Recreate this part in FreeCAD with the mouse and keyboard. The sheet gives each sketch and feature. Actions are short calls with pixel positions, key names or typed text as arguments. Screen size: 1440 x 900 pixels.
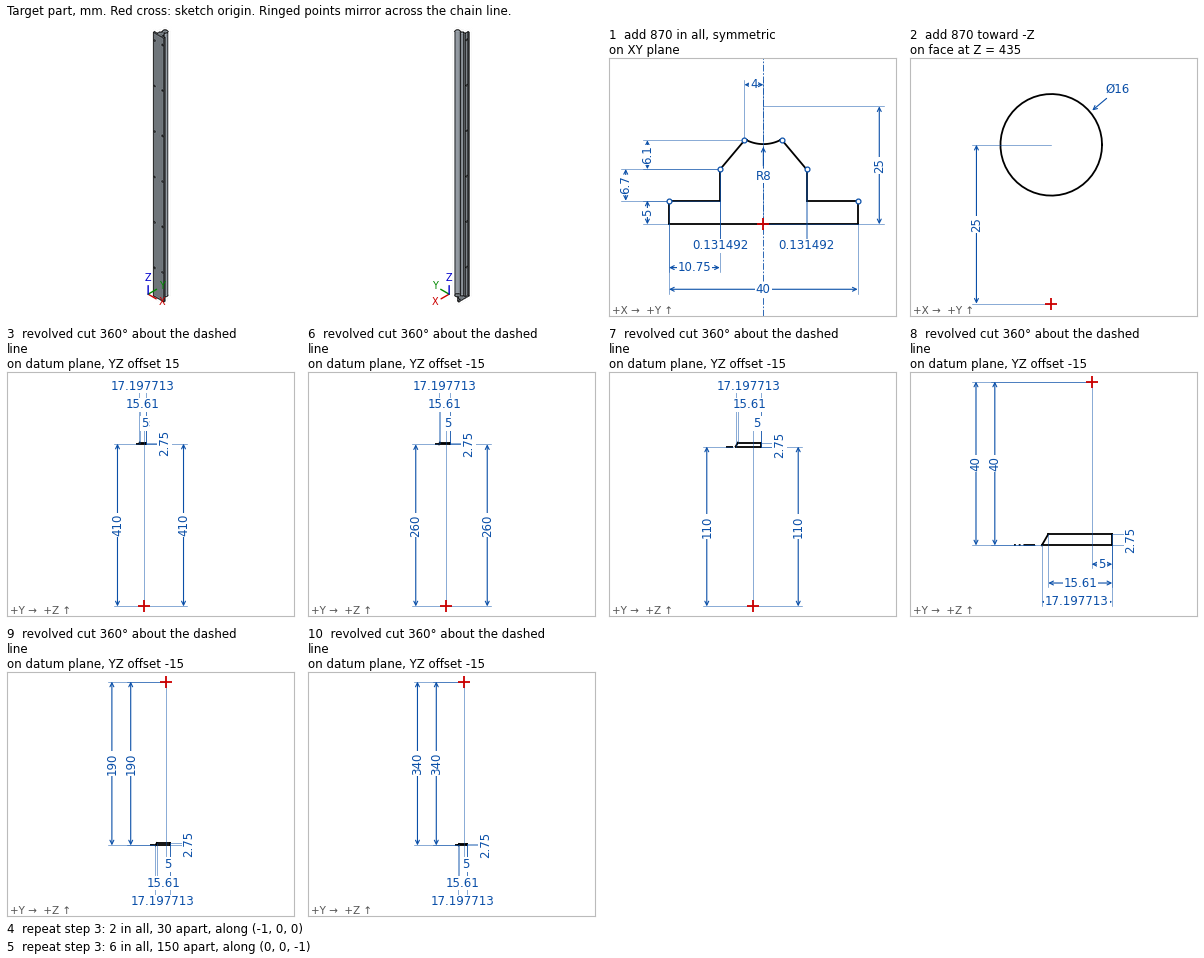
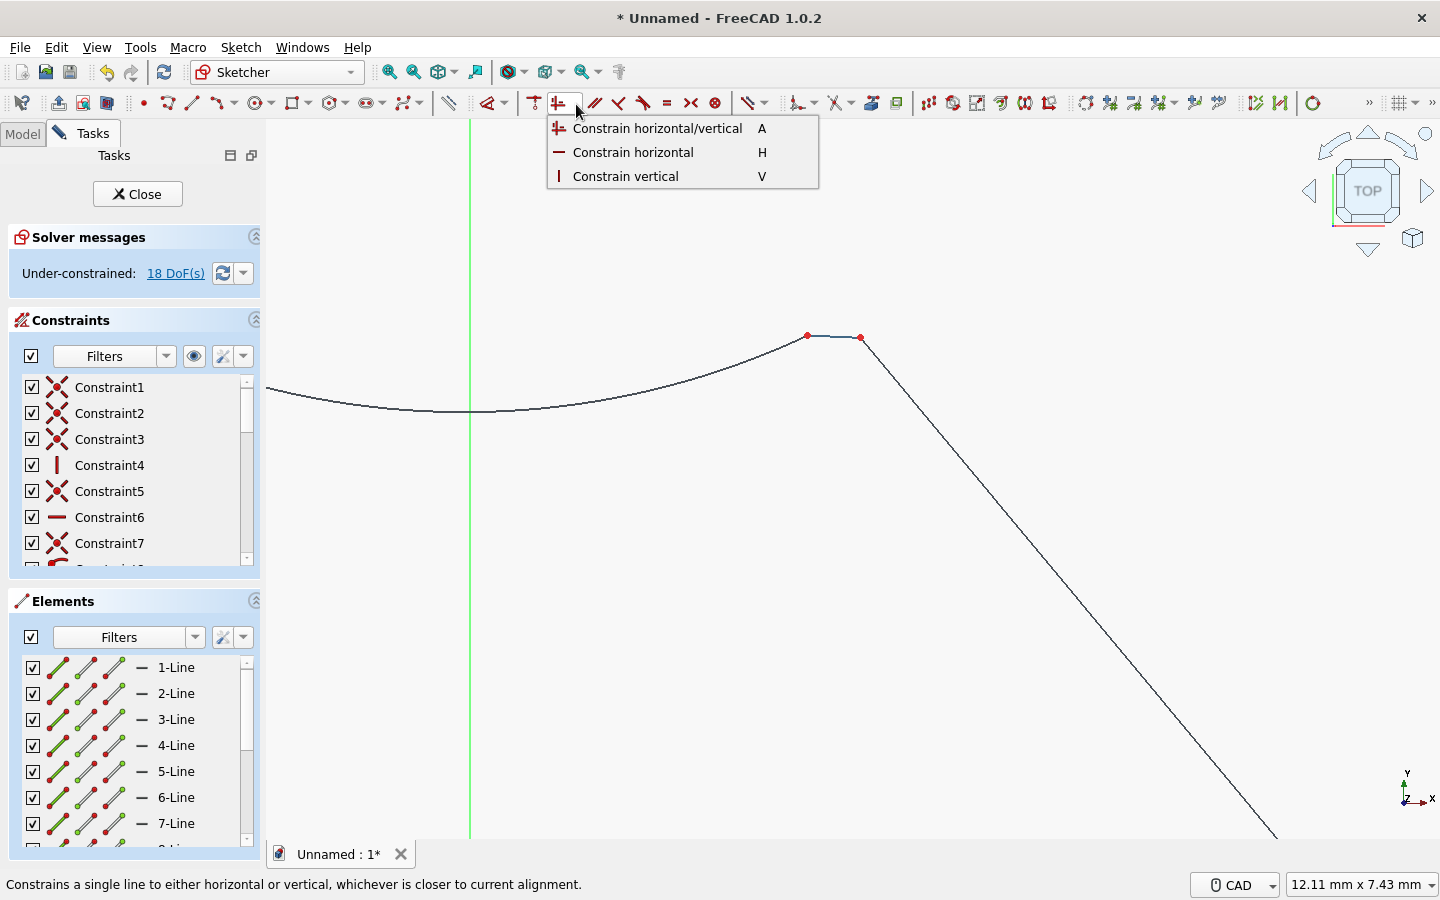
click(683, 152)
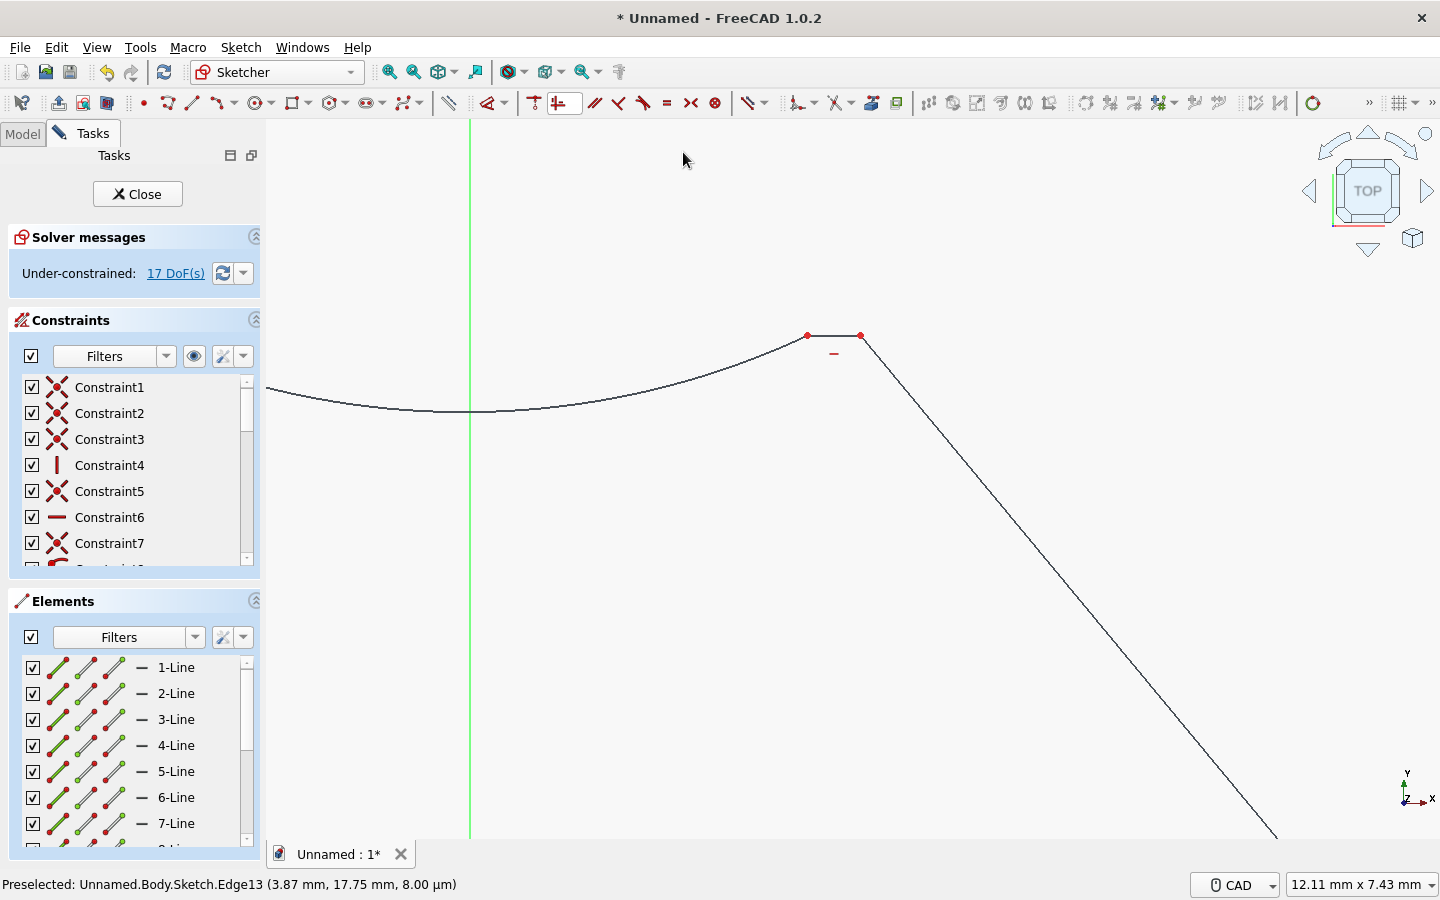
scroll(847, 337, down, 9)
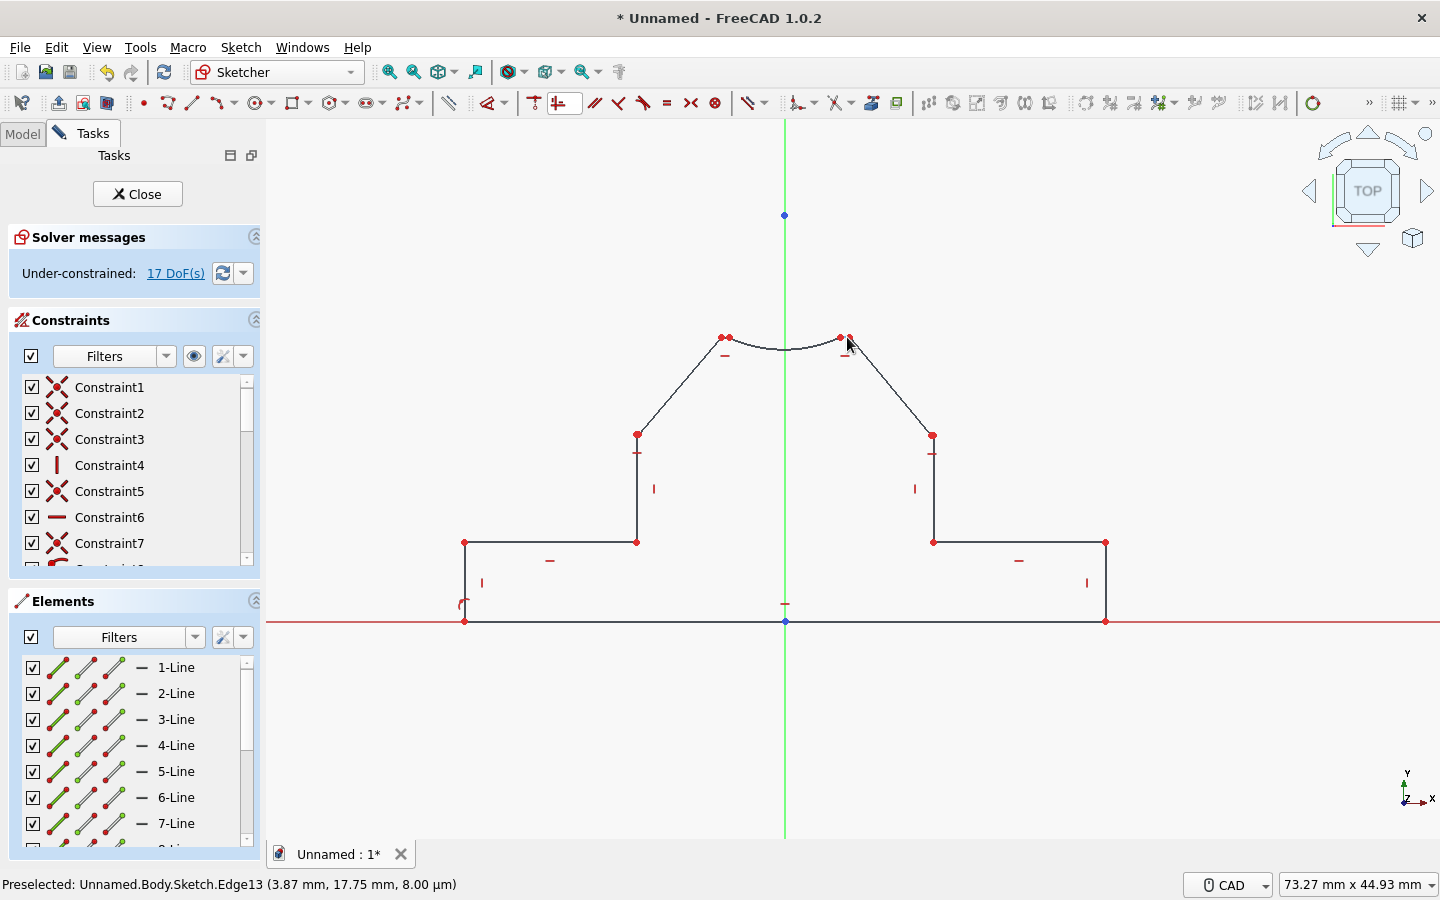
click(784, 216)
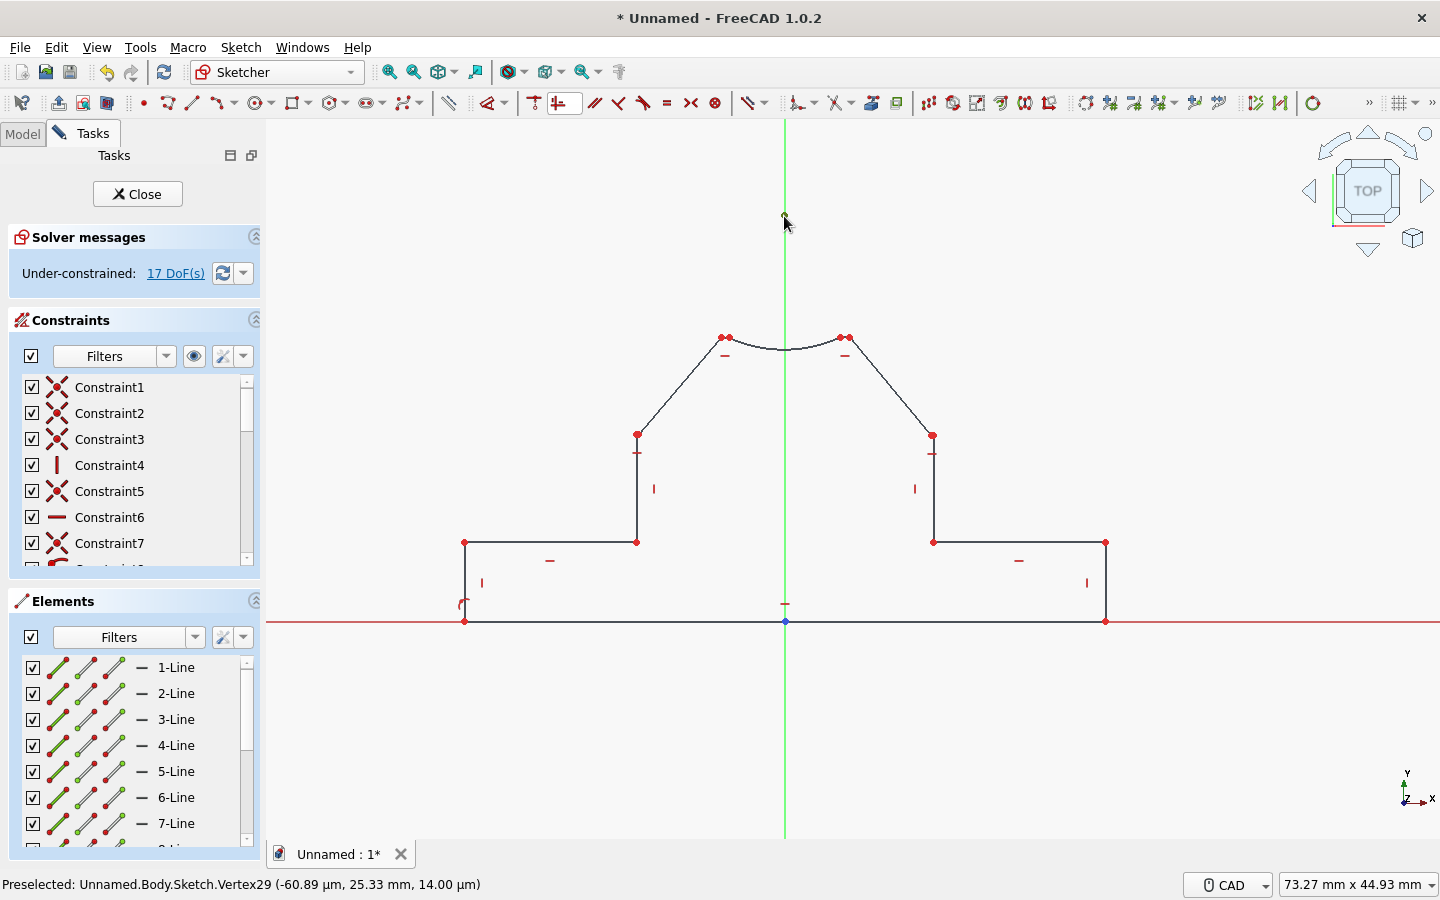
click(785, 764)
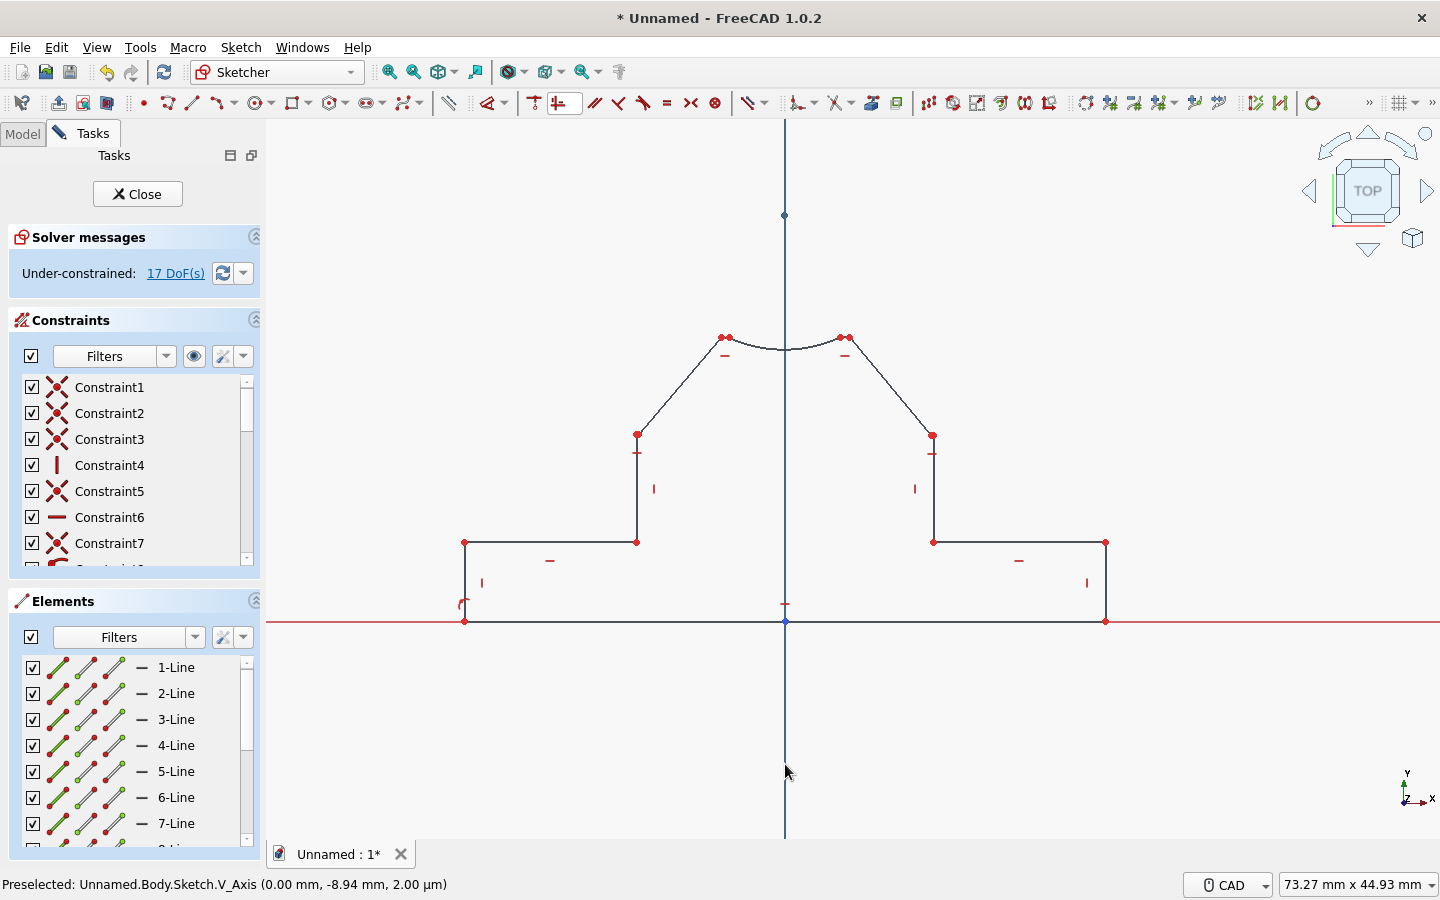
key(c)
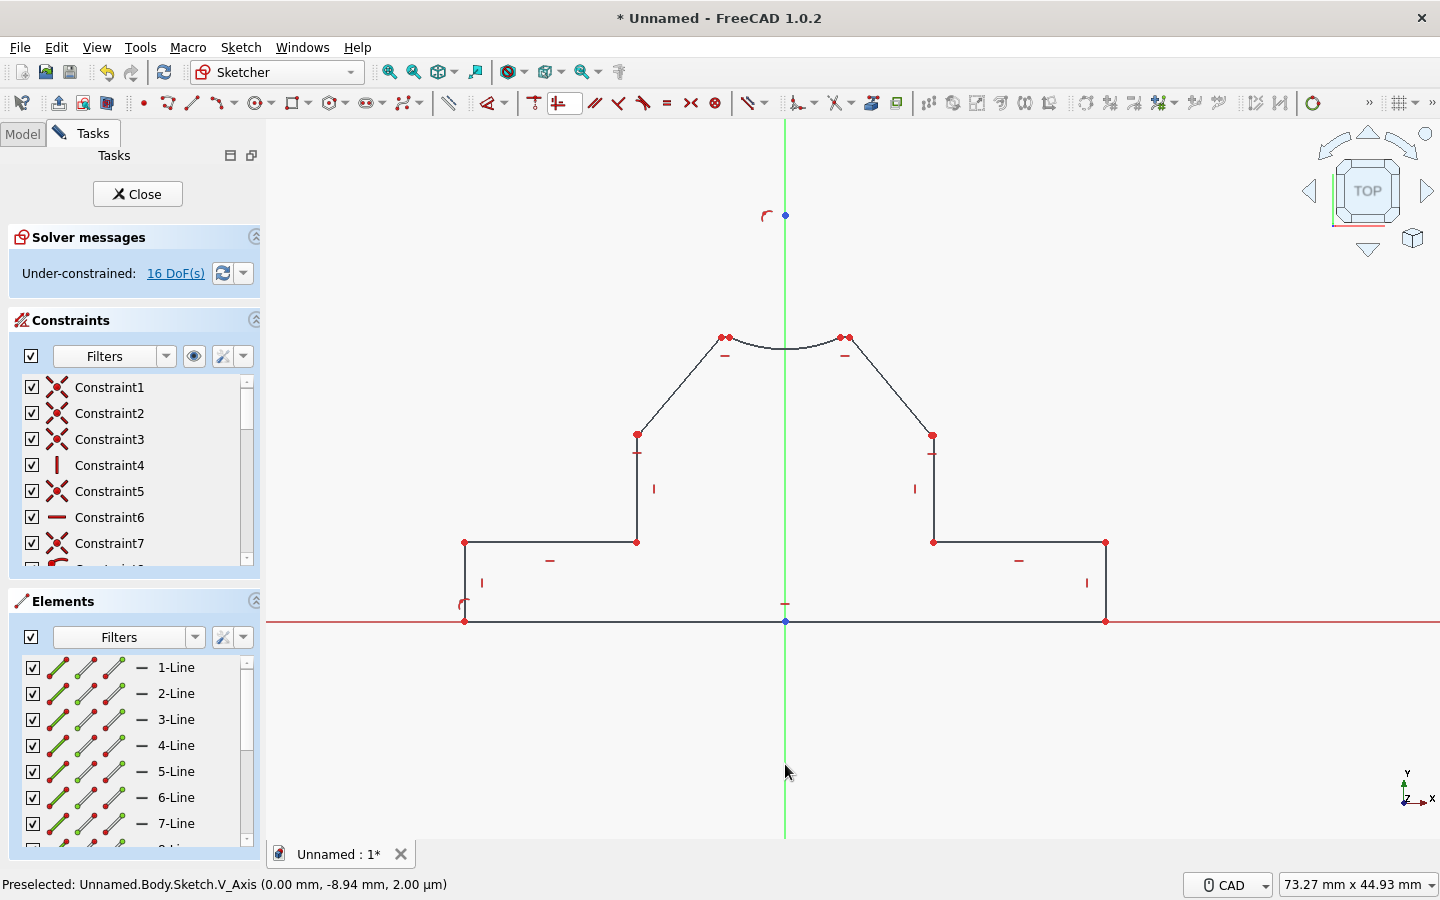
click(465, 542)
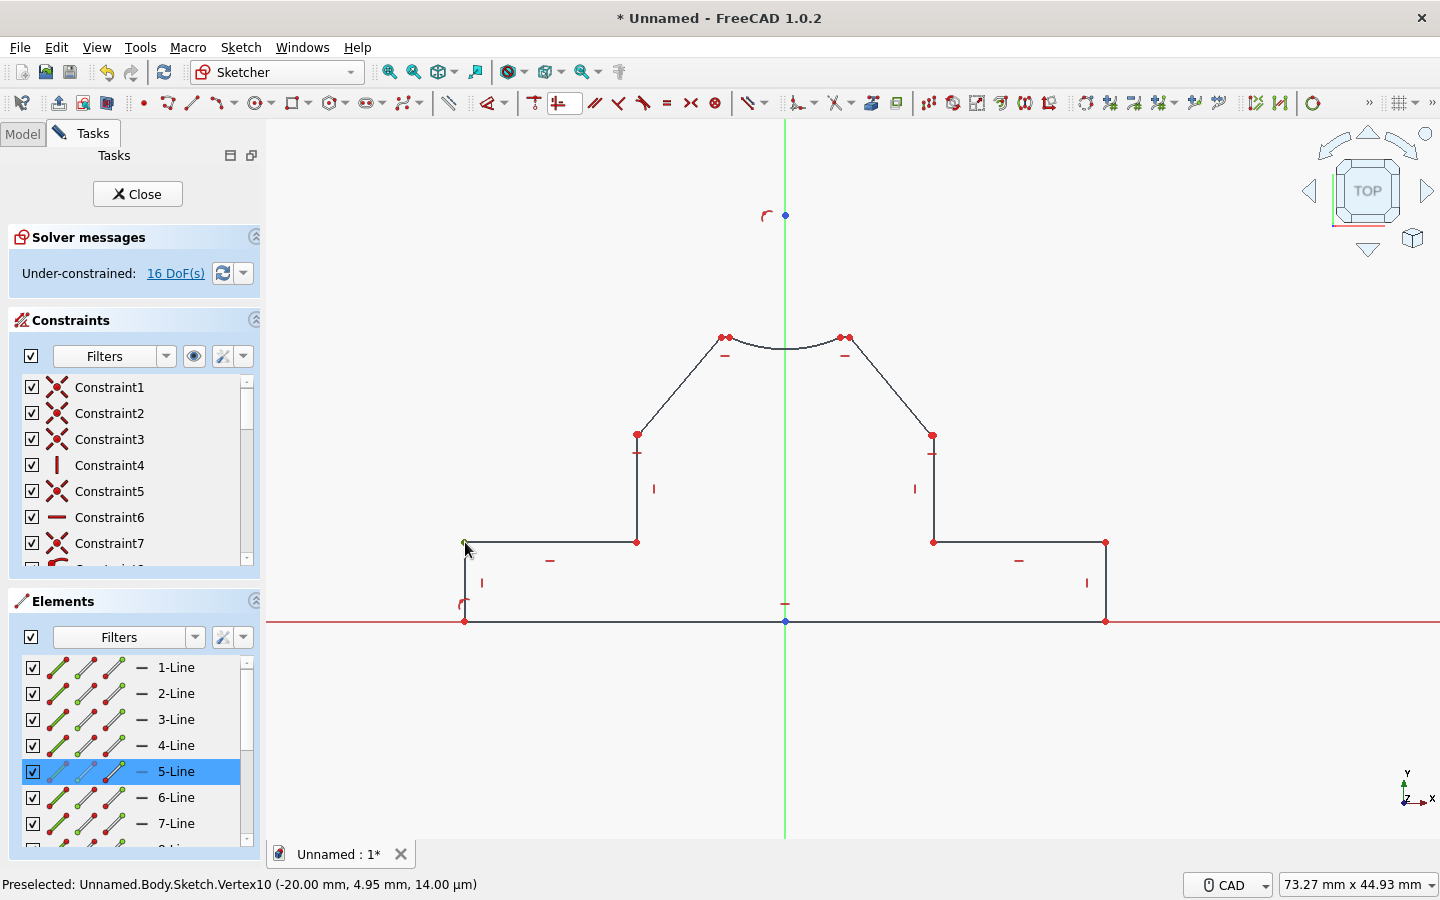
click(1106, 542)